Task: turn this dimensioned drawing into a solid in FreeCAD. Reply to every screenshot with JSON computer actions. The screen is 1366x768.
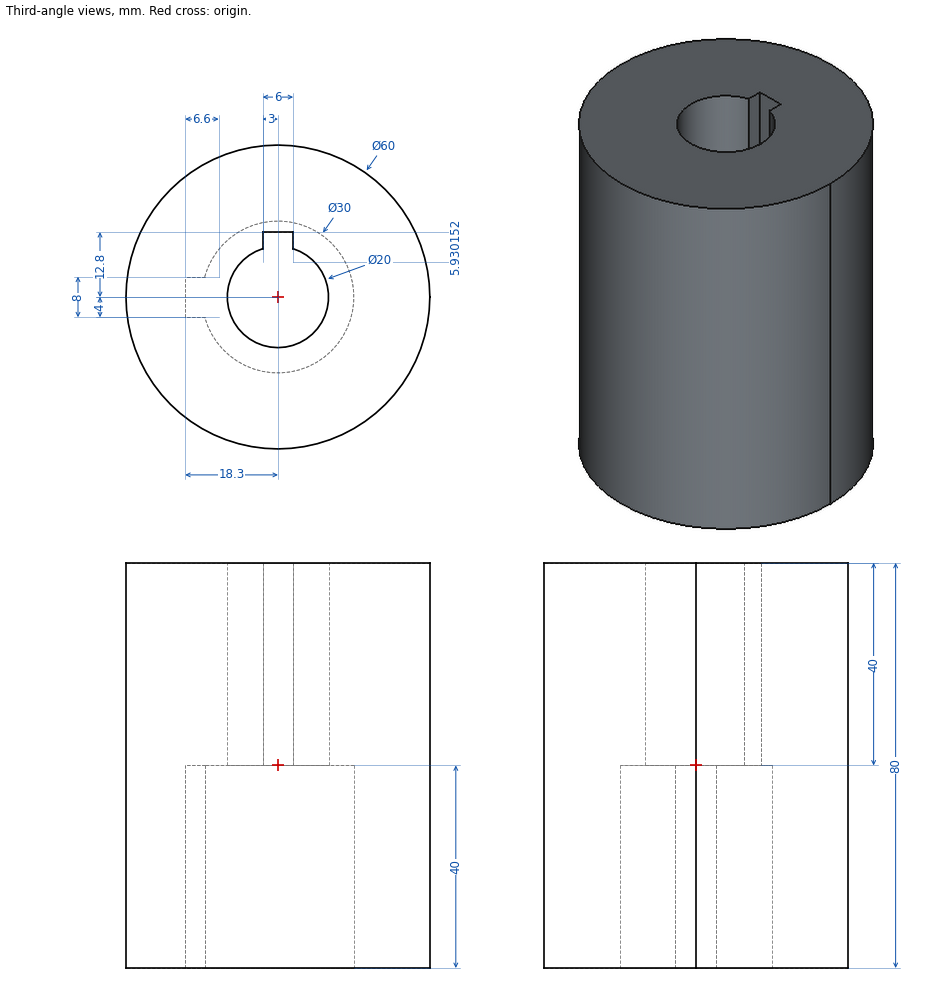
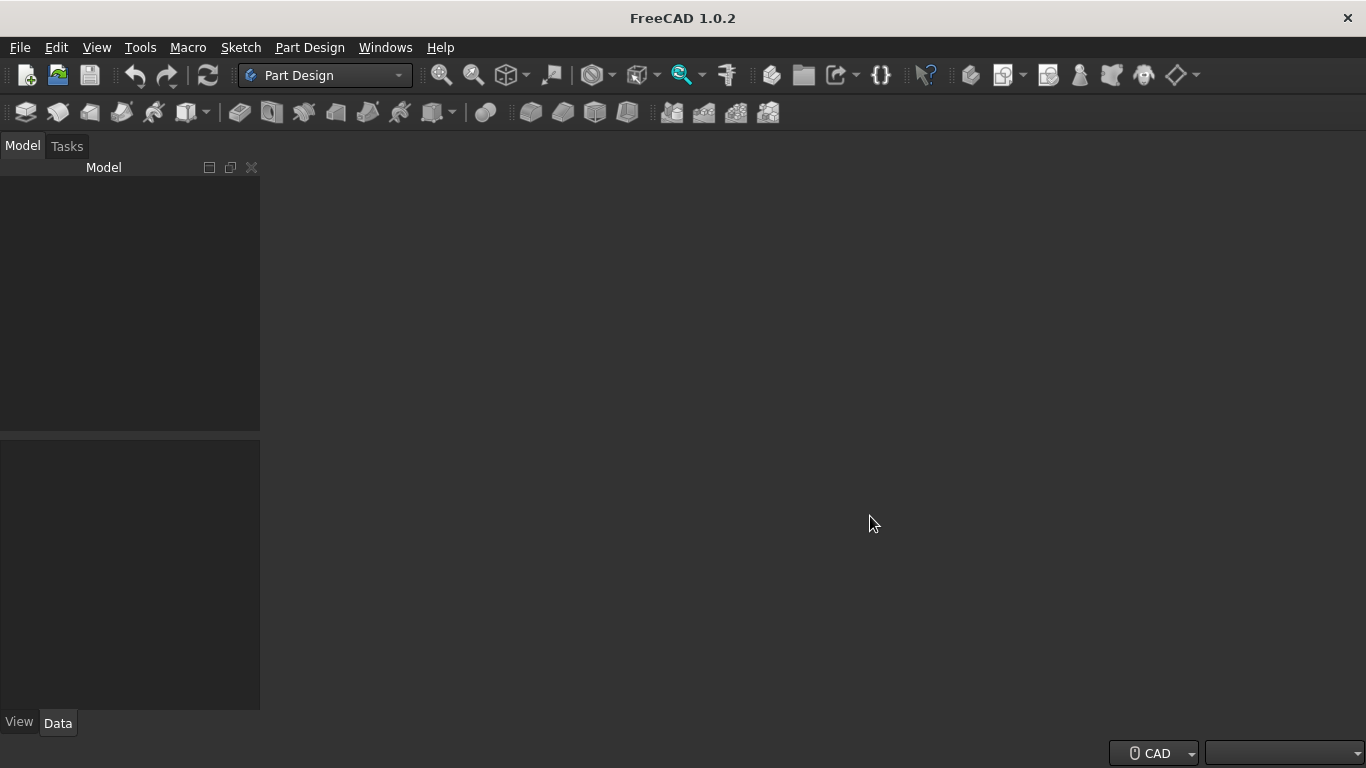
{"action": "key", "text": "ctrl+n"}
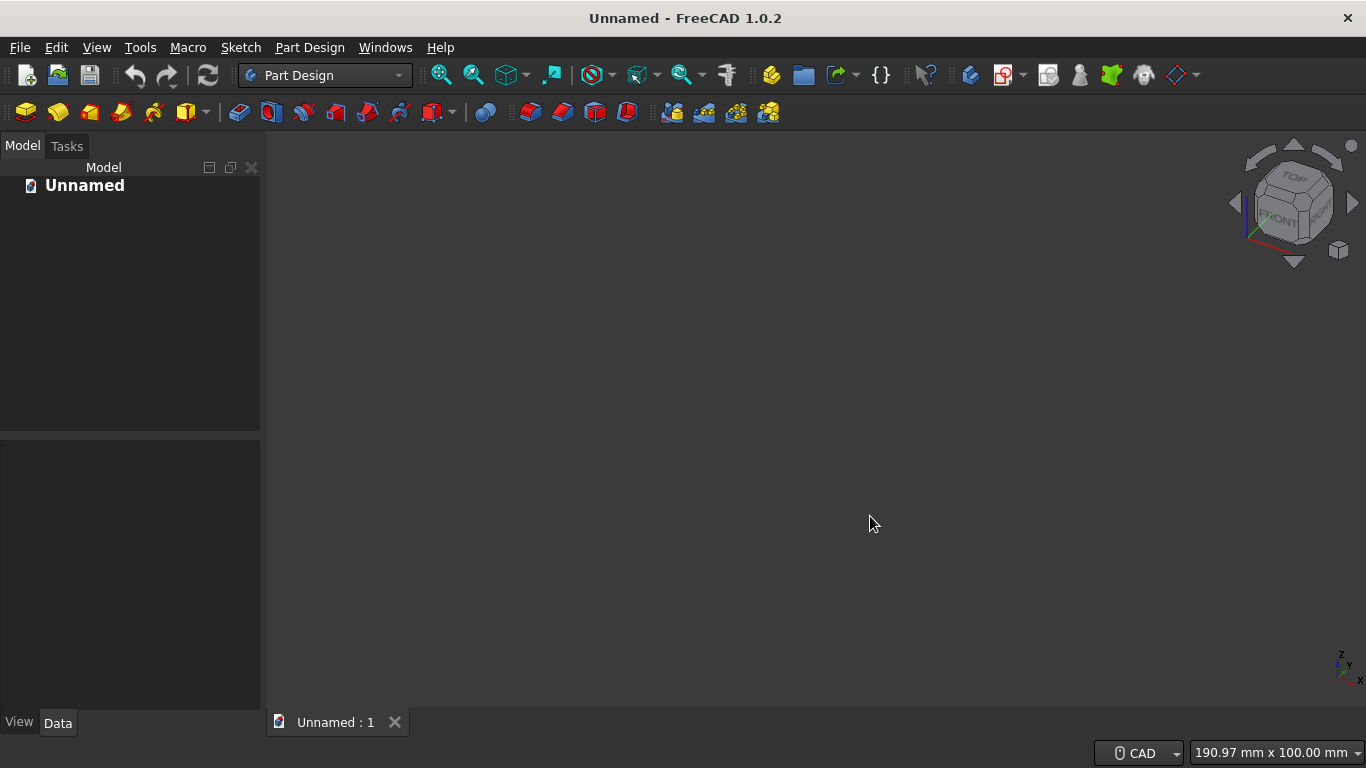
{"action": "left_click", "coordinate": [1004, 76]}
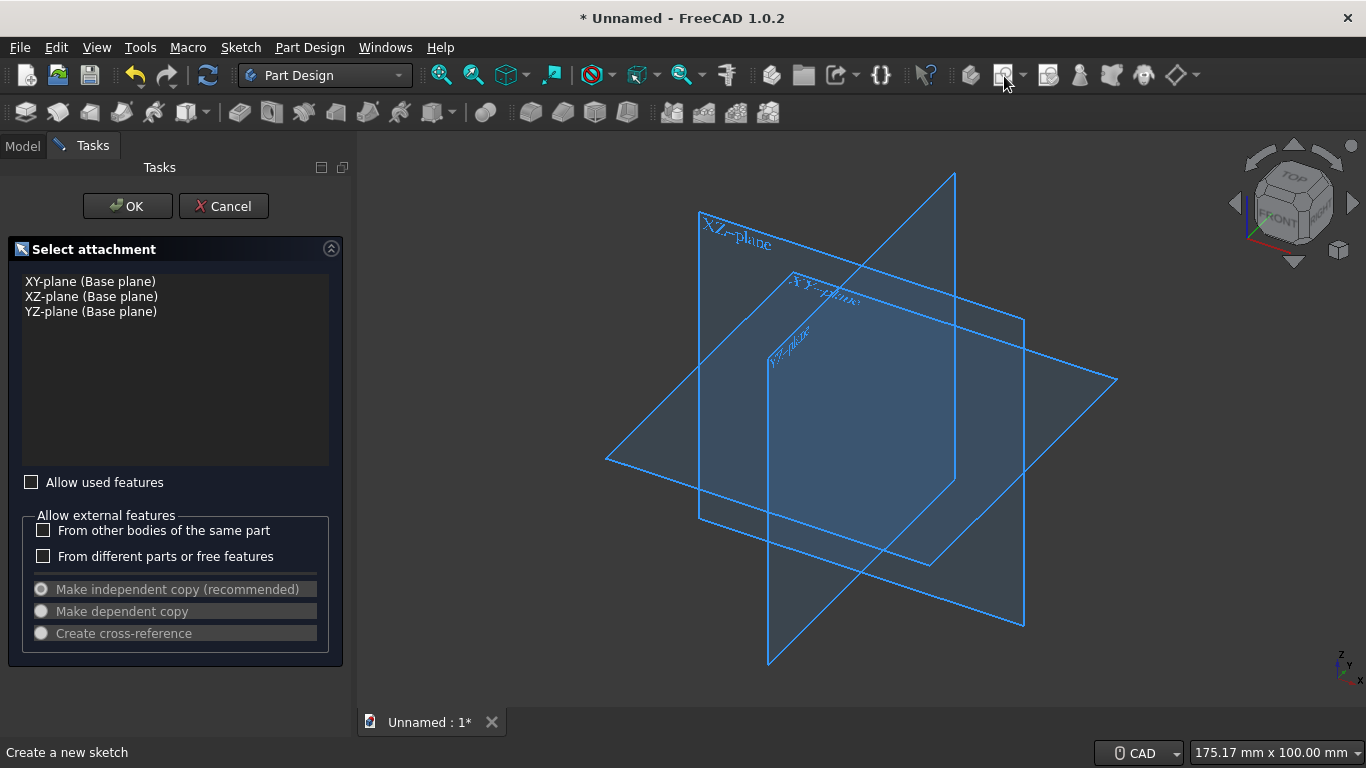
{"action": "left_click", "coordinate": [82, 282]}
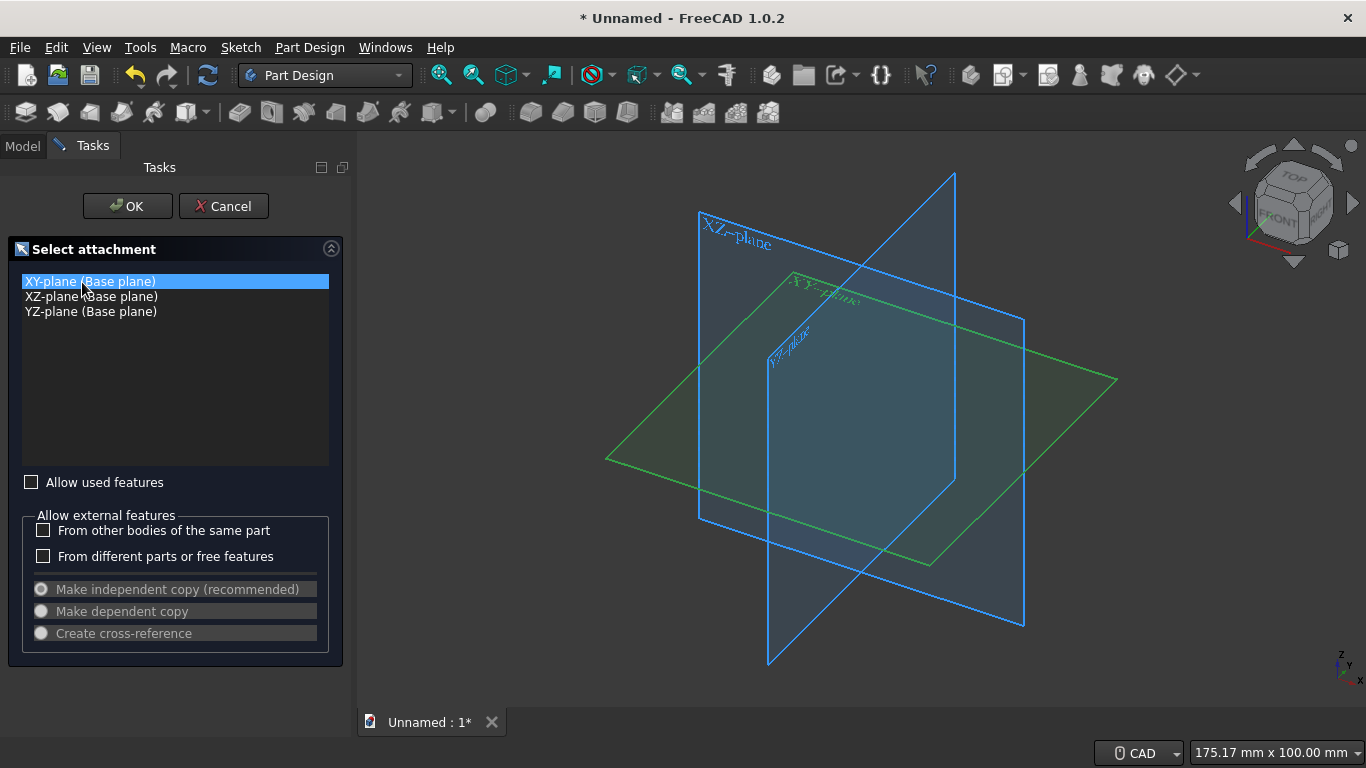
{"action": "left_click", "coordinate": [128, 206]}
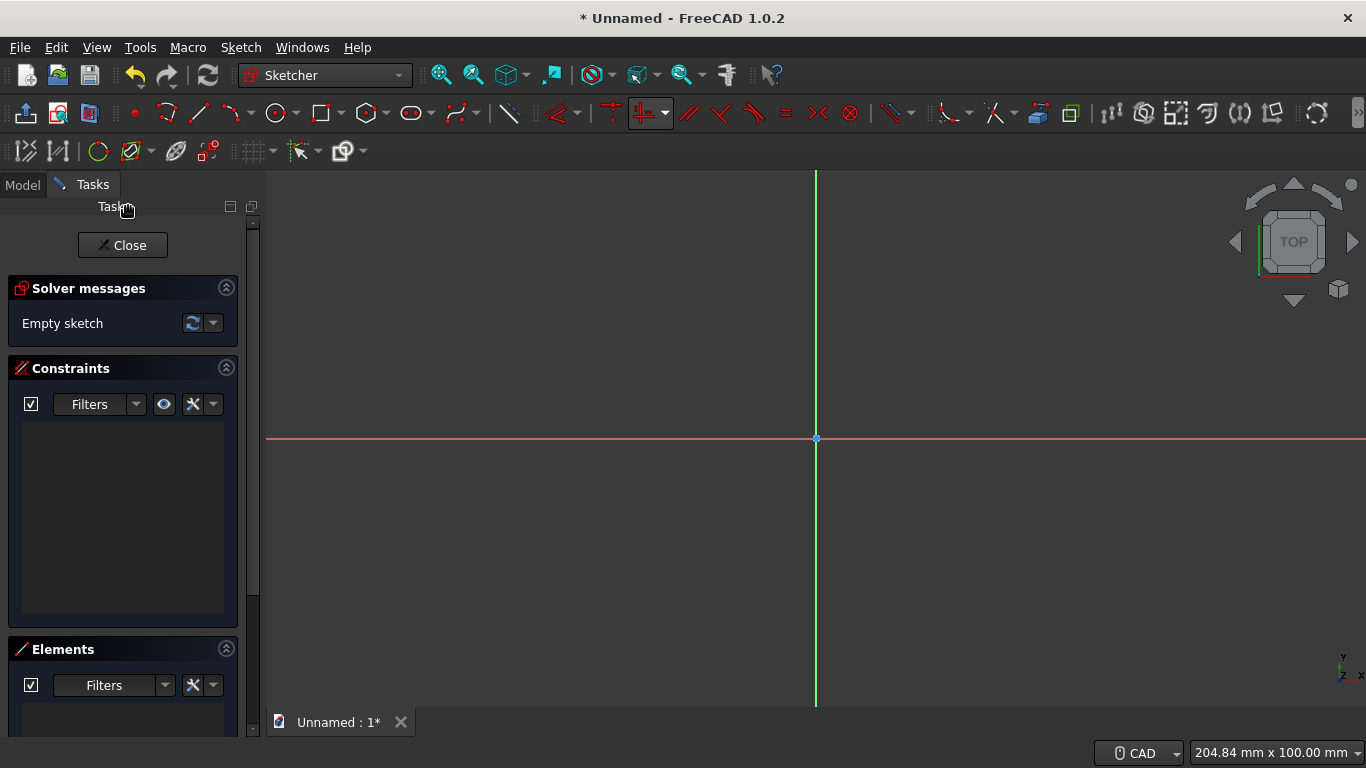
{"action": "left_click", "coordinate": [276, 114]}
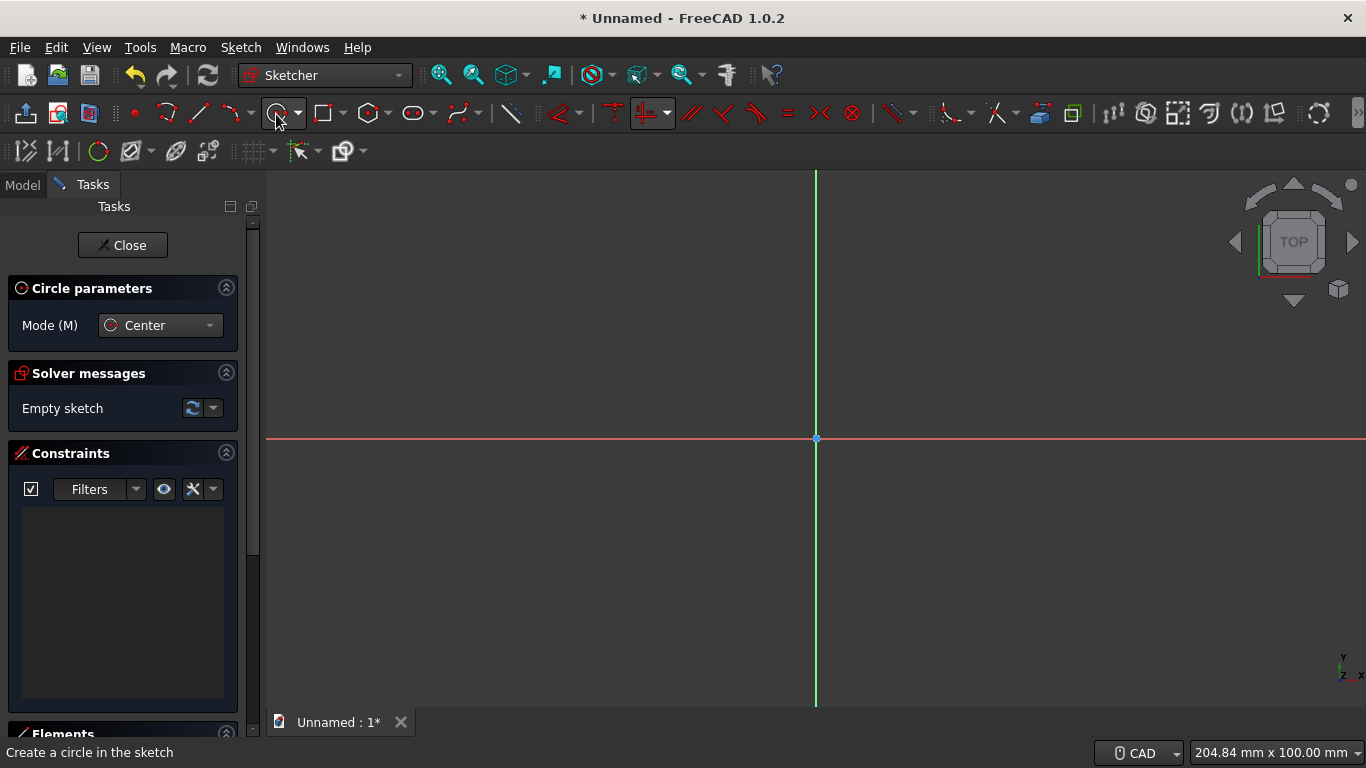
{"action": "left_click", "coordinate": [816, 438]}
{"action": "mouse_move", "coordinate": [930, 325]}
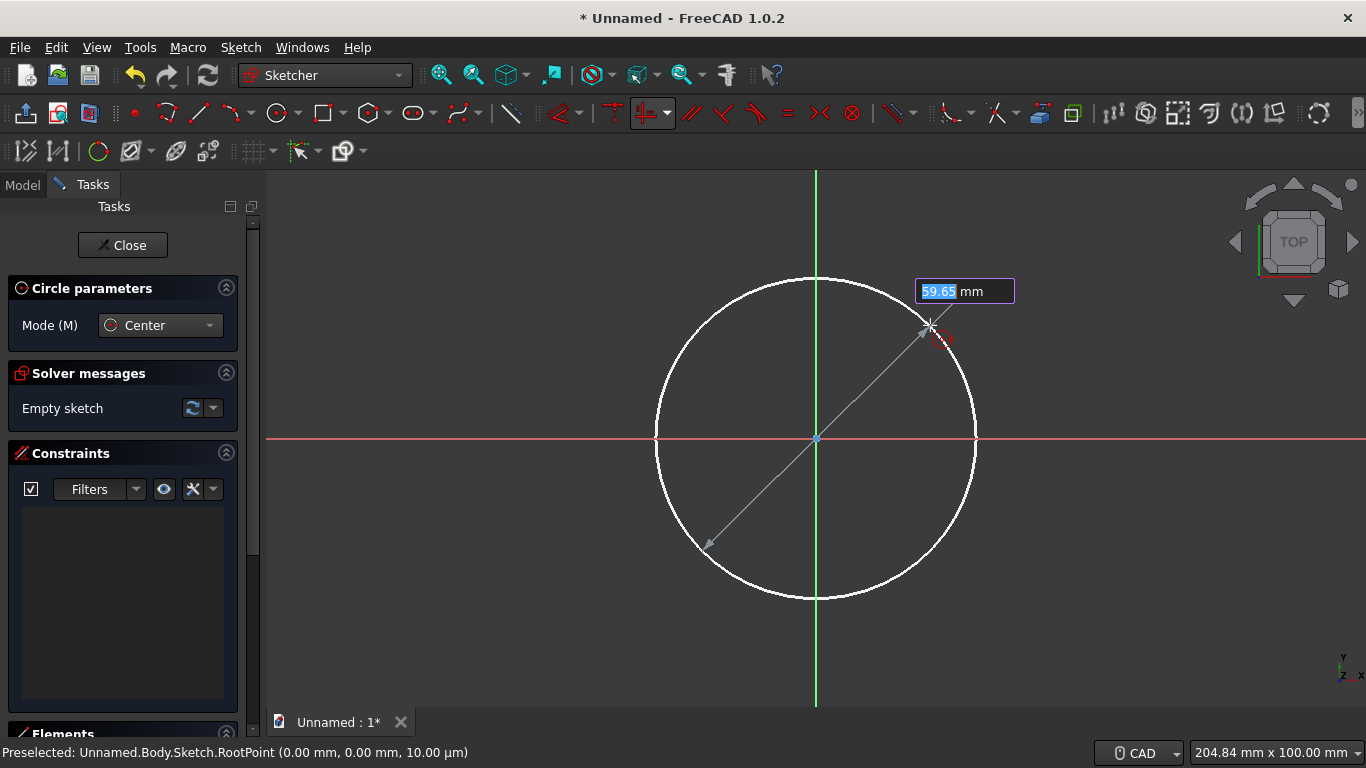
{"action": "type", "text": "60"}
{"action": "key", "text": "Return"}
{"action": "key", "text": "Escape"}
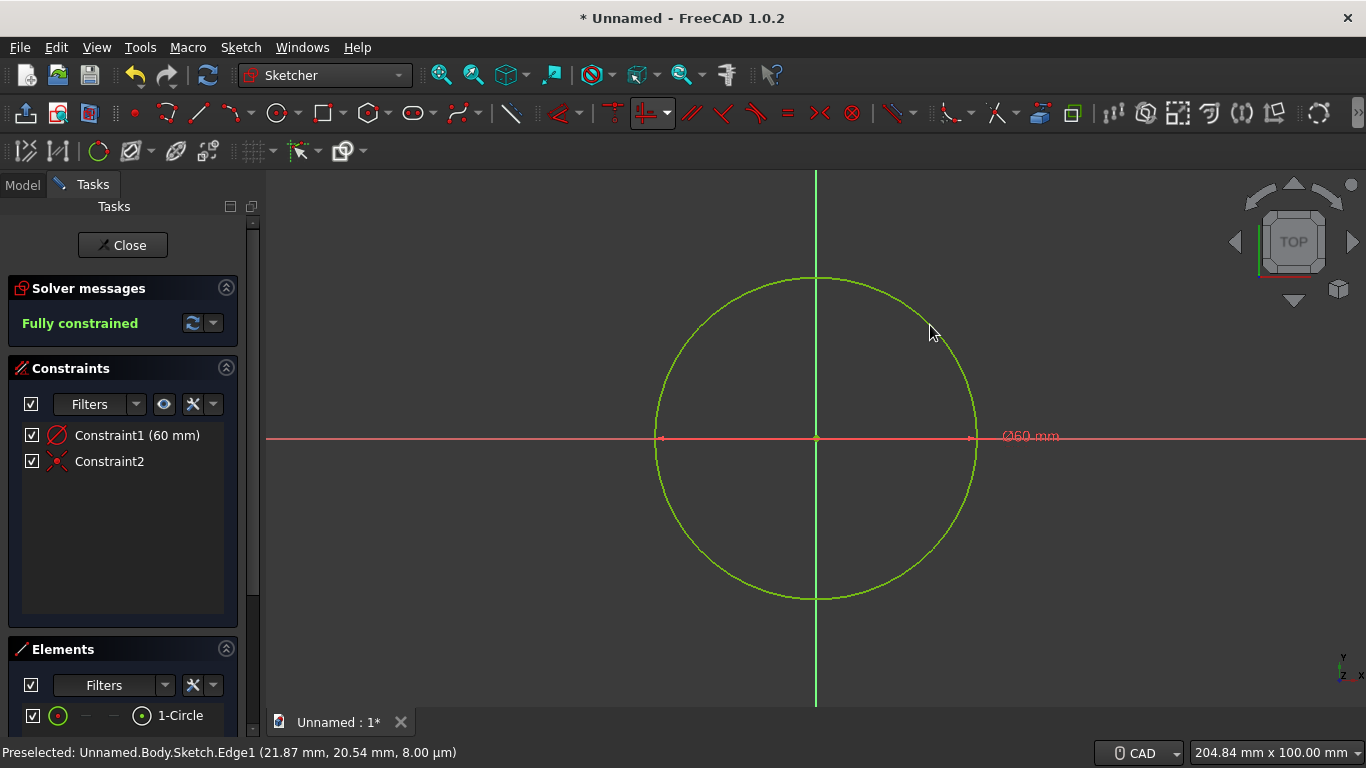
{"action": "left_click", "coordinate": [123, 245]}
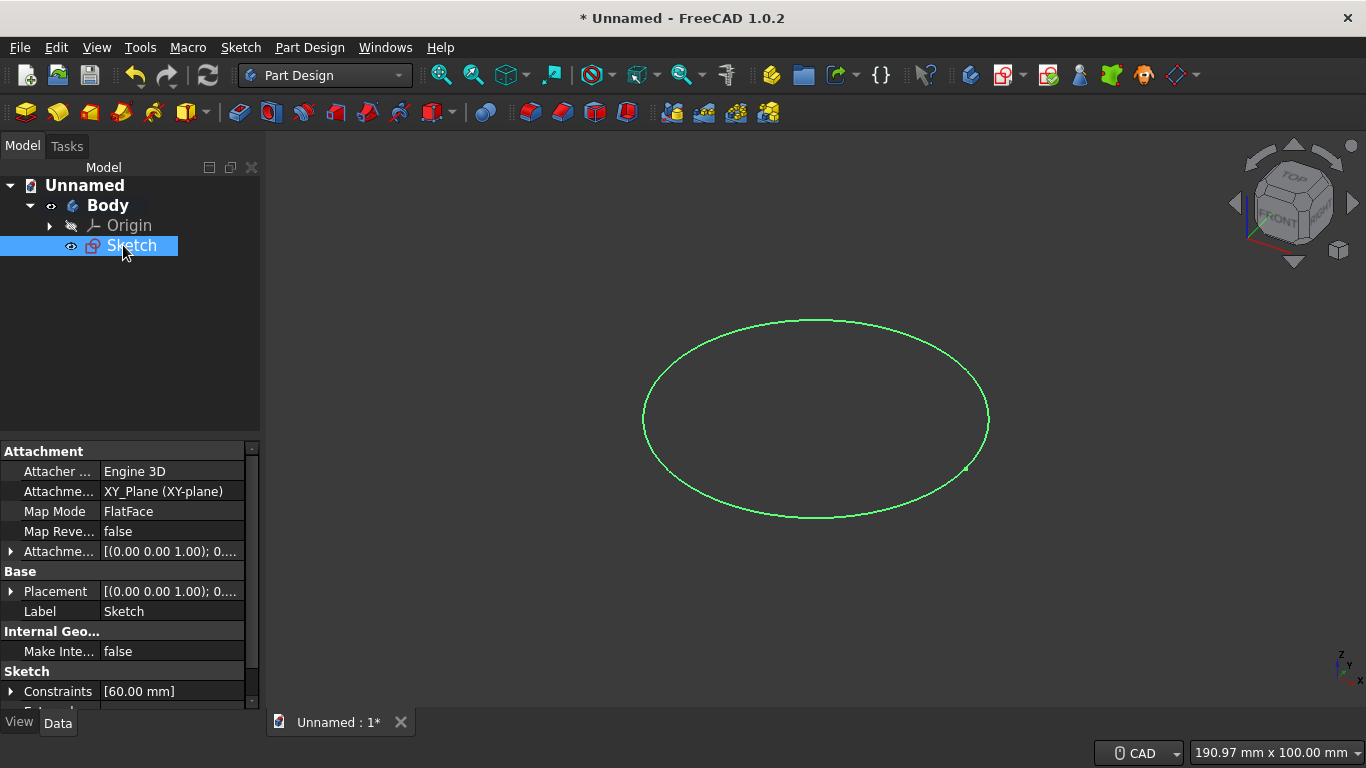
{"action": "left_click", "coordinate": [26, 112]}